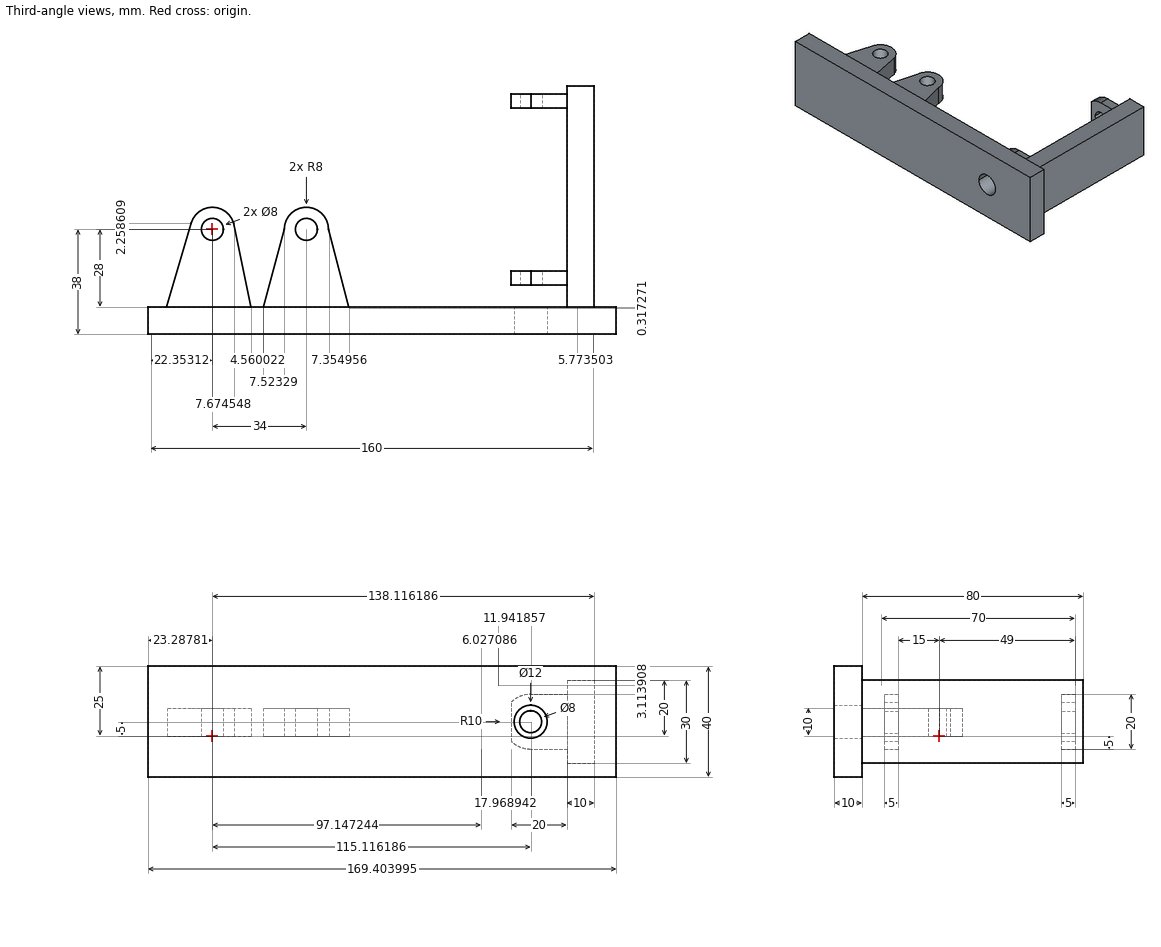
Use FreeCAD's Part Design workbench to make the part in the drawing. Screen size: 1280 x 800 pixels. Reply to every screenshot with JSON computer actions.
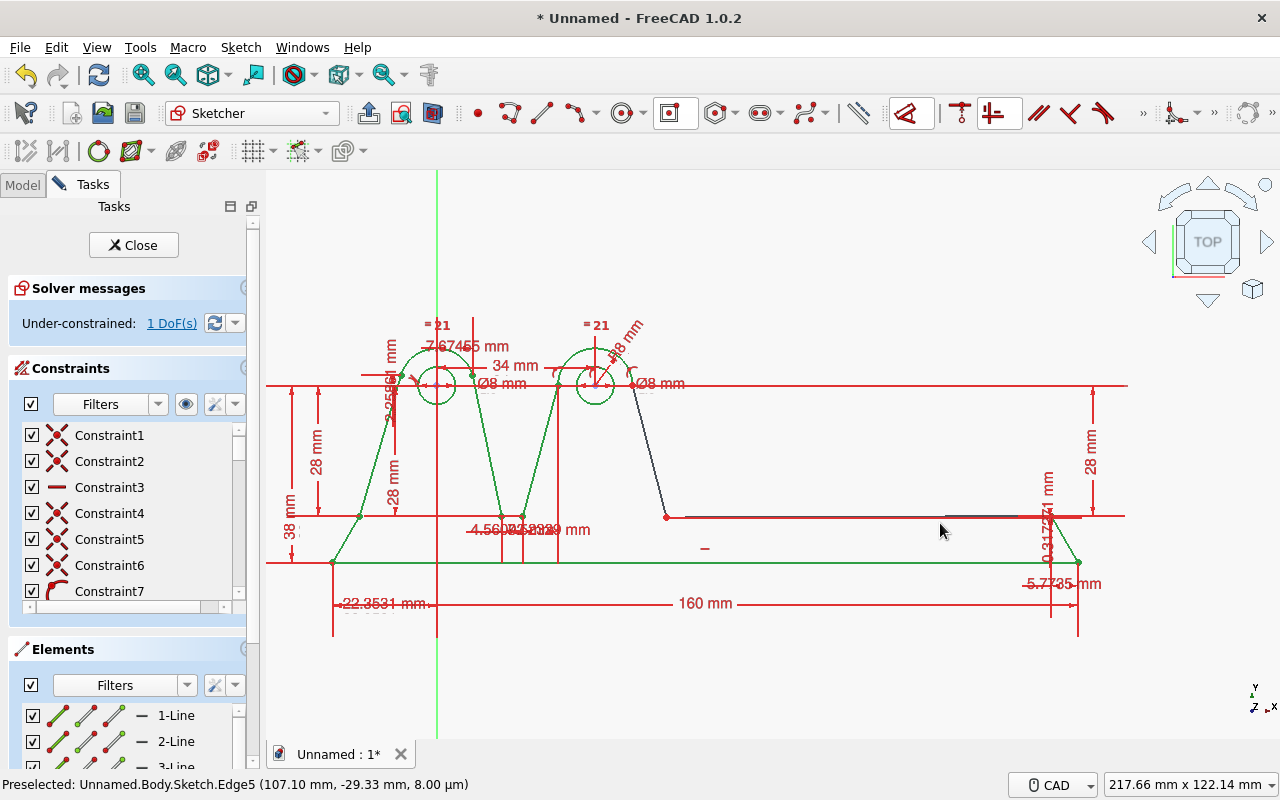
{"action": "left_click", "coordinate": [656, 478]}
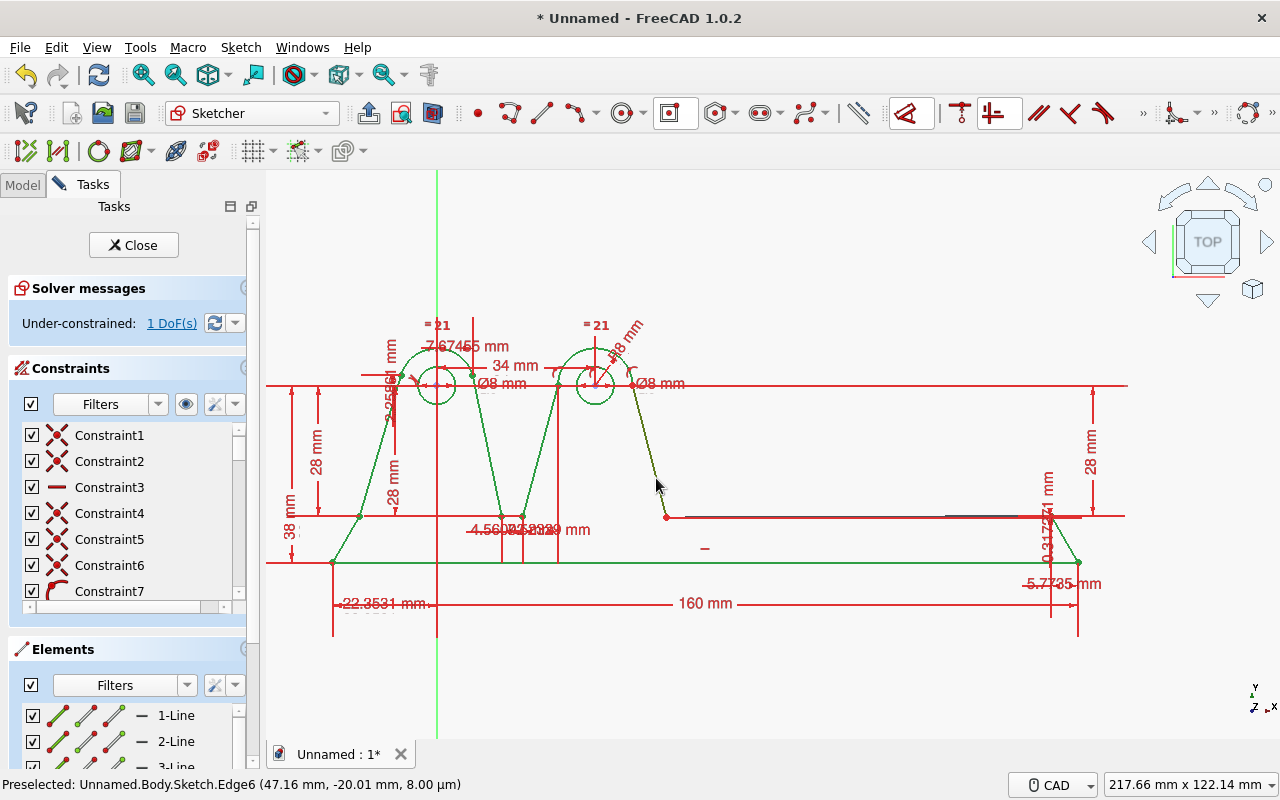
{"action": "left_click", "coordinate": [928, 114]}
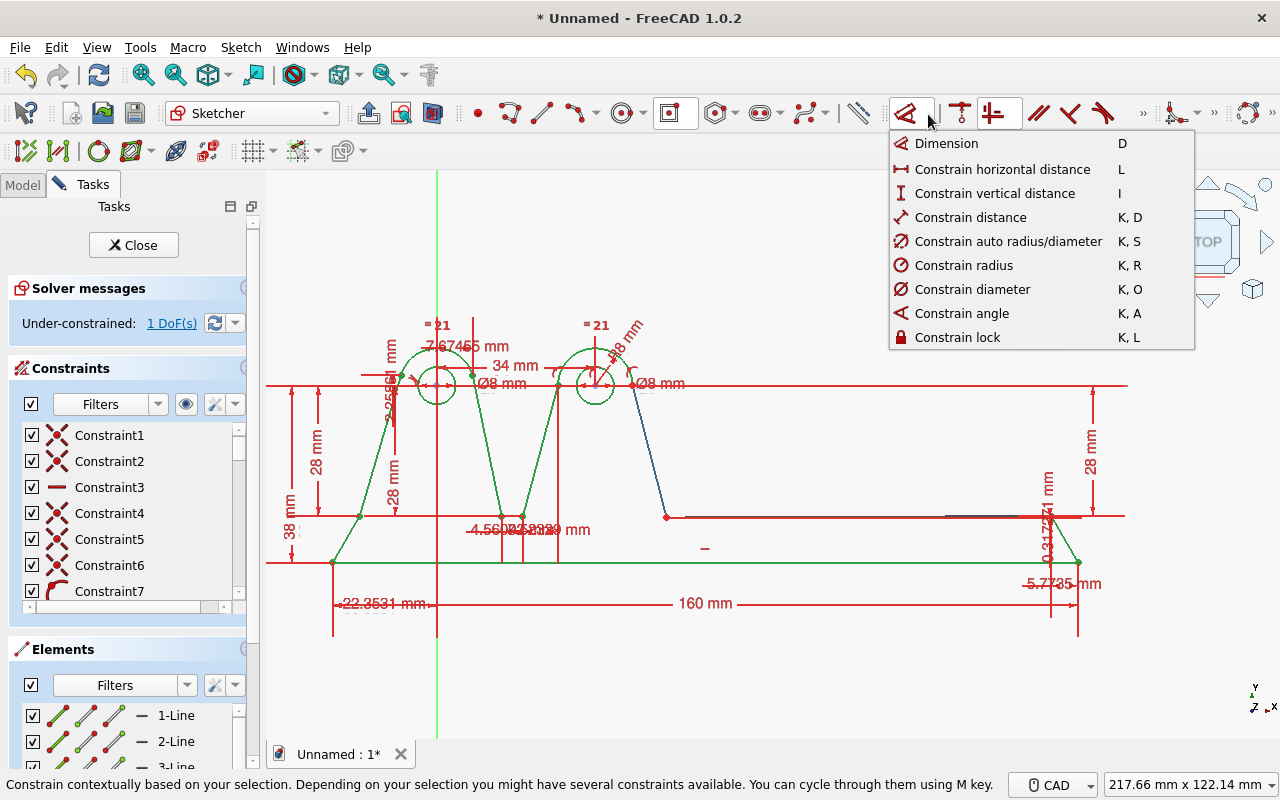
{"action": "left_click", "coordinate": [1042, 169]}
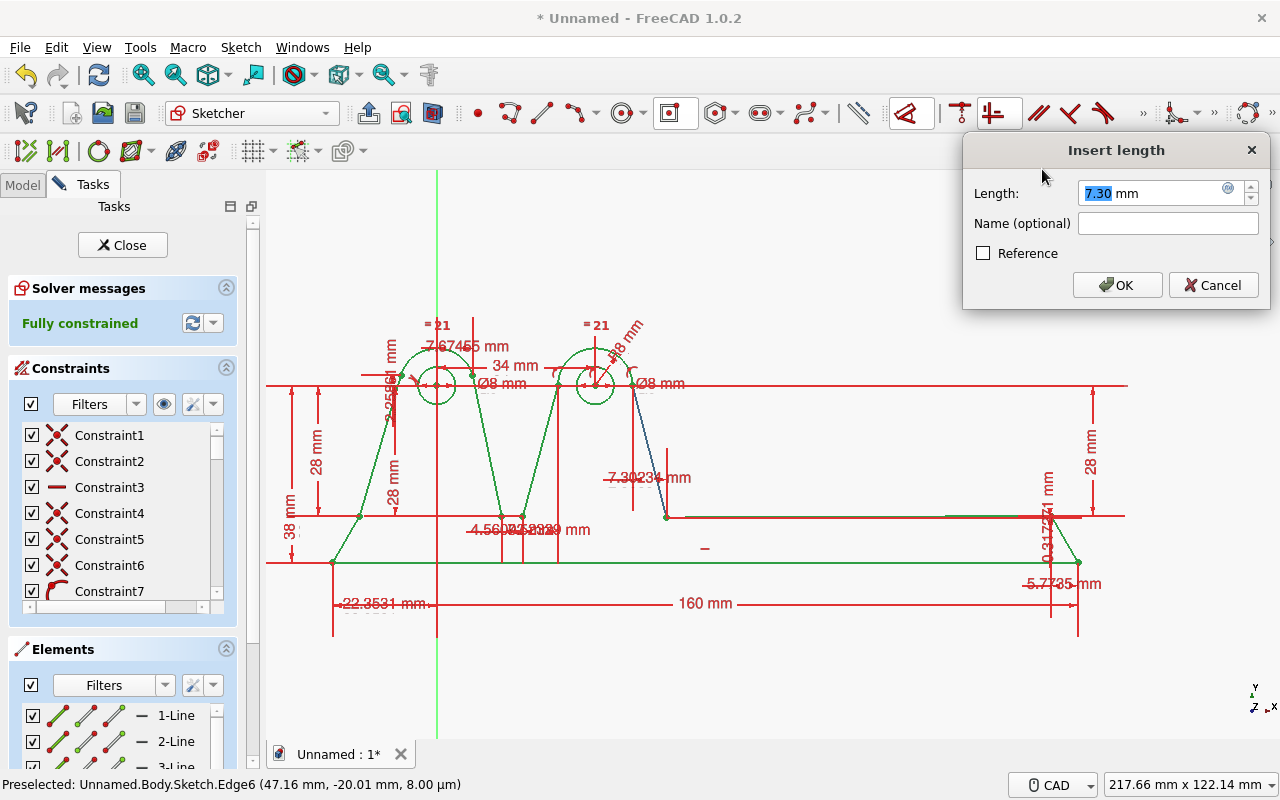
{"action": "type", "text": "7.354956"}
{"action": "key", "text": "Return"}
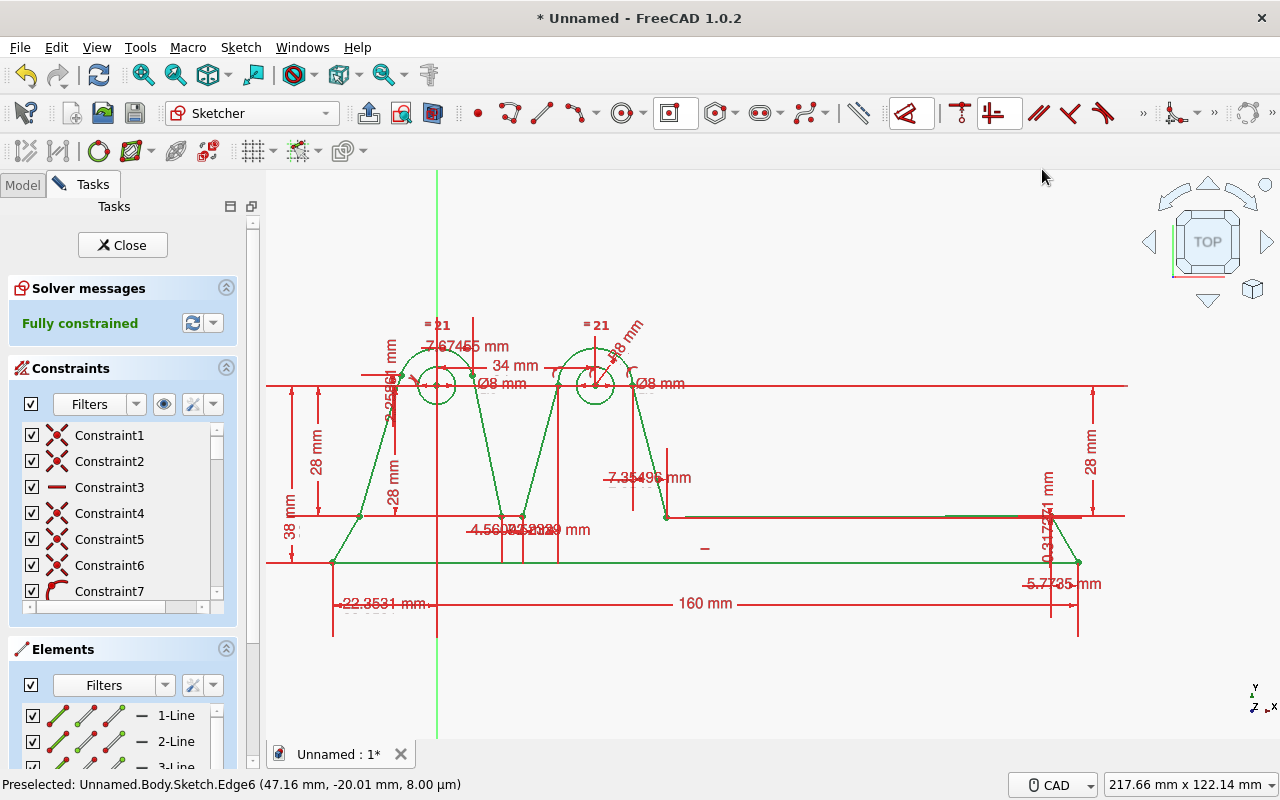
{"action": "left_click", "coordinate": [123, 245]}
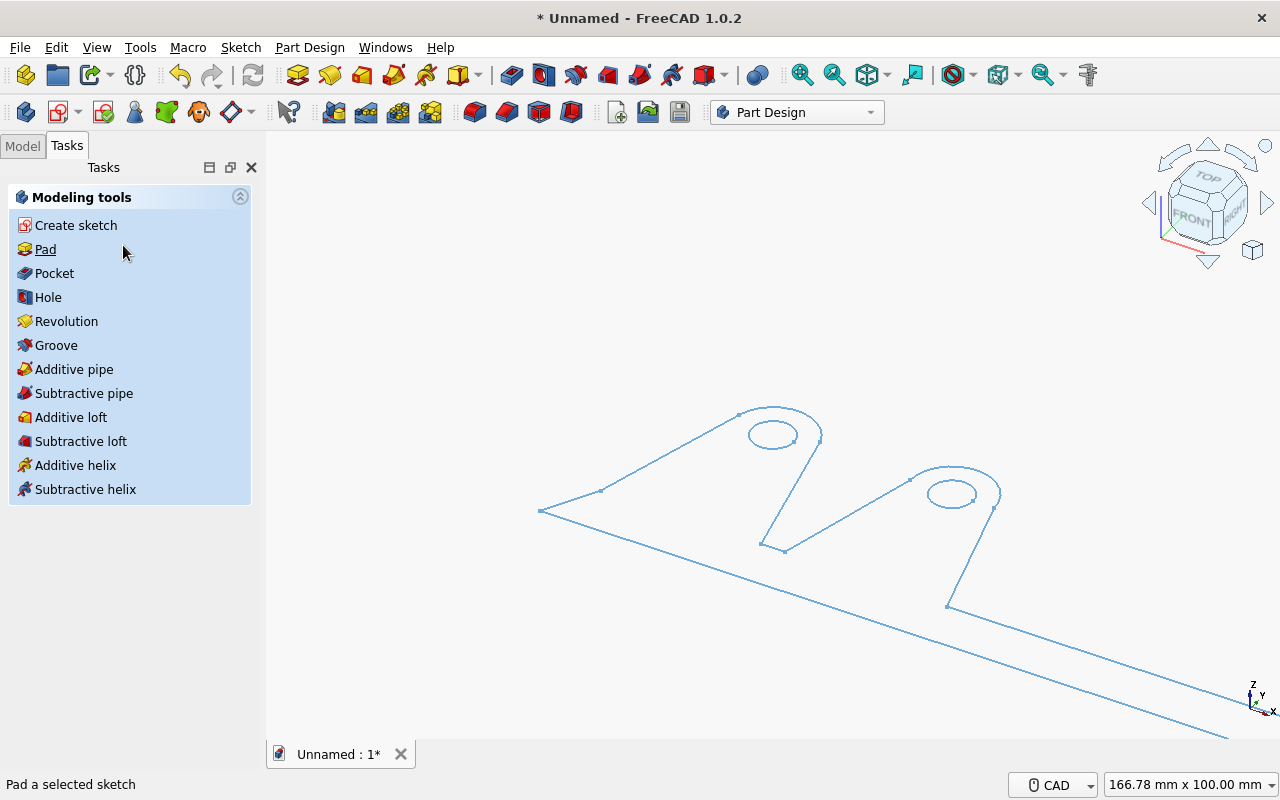
{"action": "left_click", "coordinate": [298, 76]}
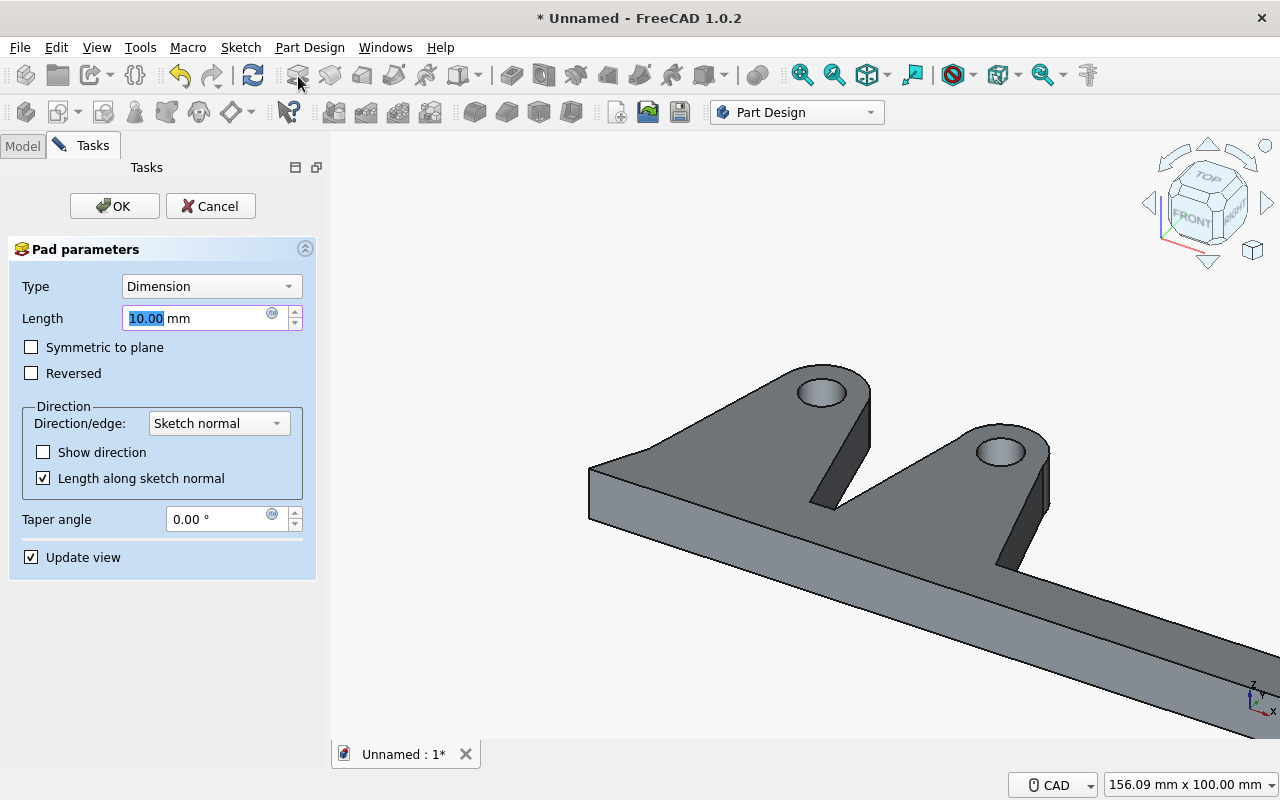
{"action": "type", "text": "10"}
{"action": "key", "text": "Tab"}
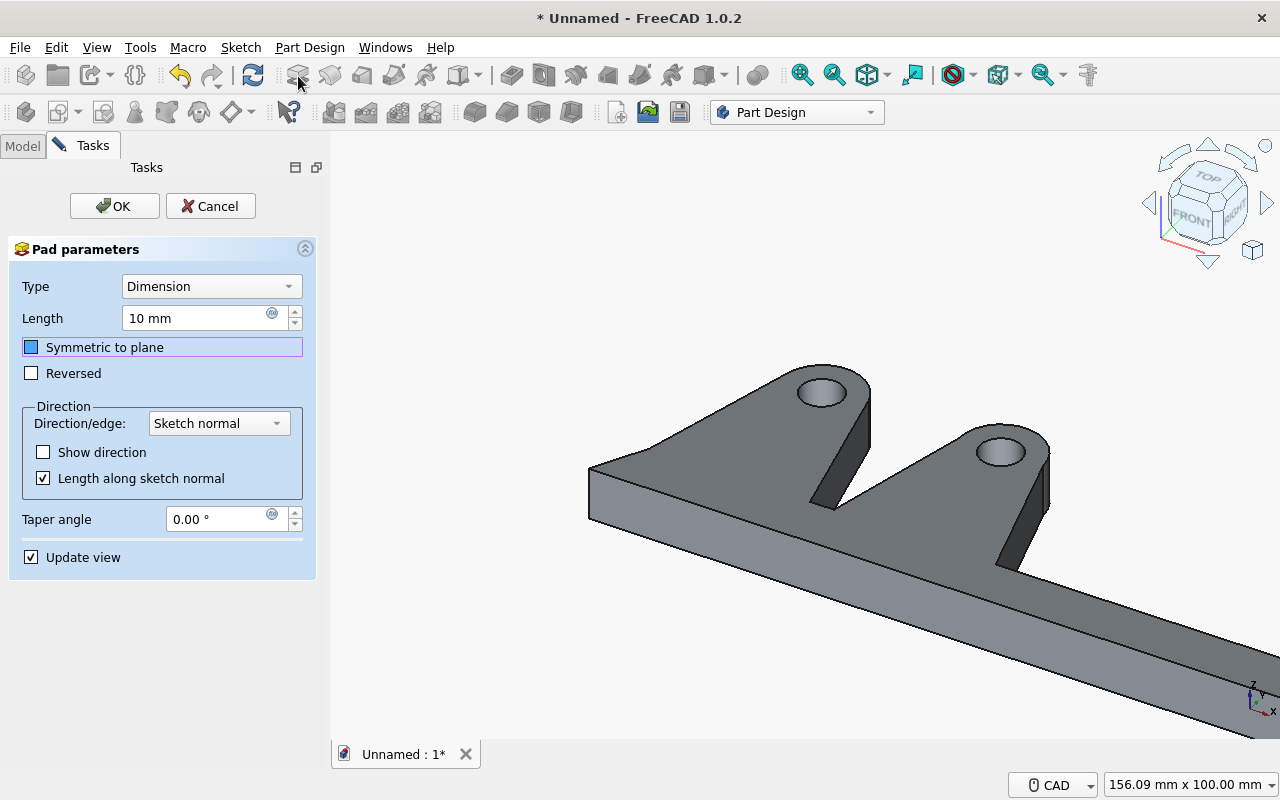
{"action": "left_click", "coordinate": [115, 206]}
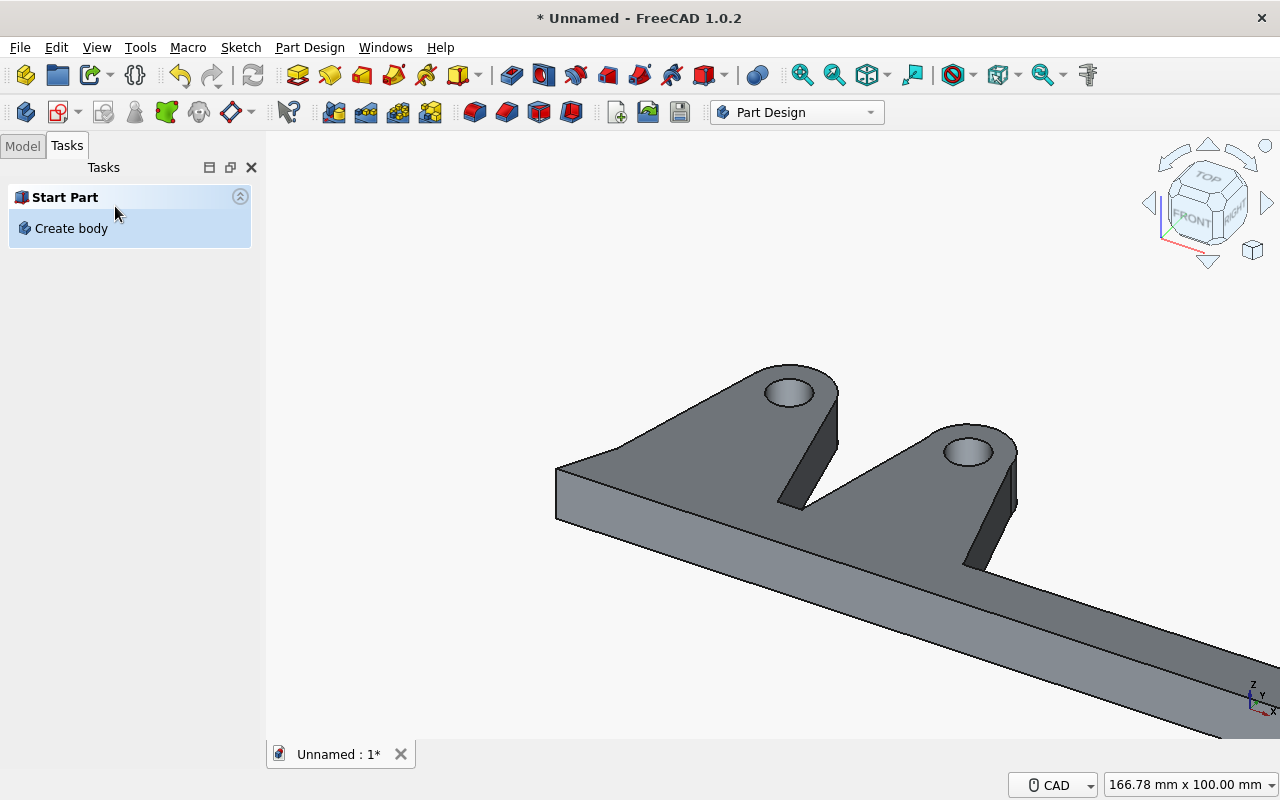
{"action": "left_click", "coordinate": [804, 76]}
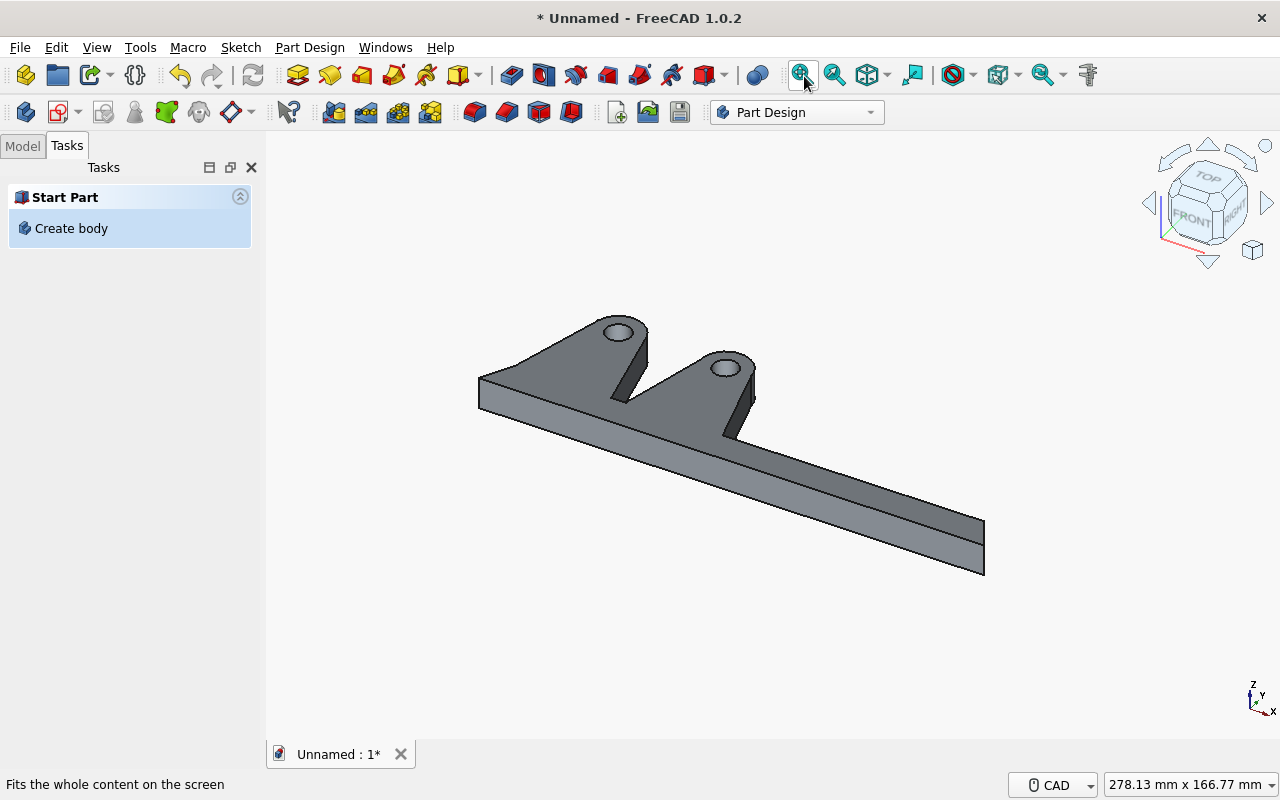
{"action": "left_click", "coordinate": [948, 547]}